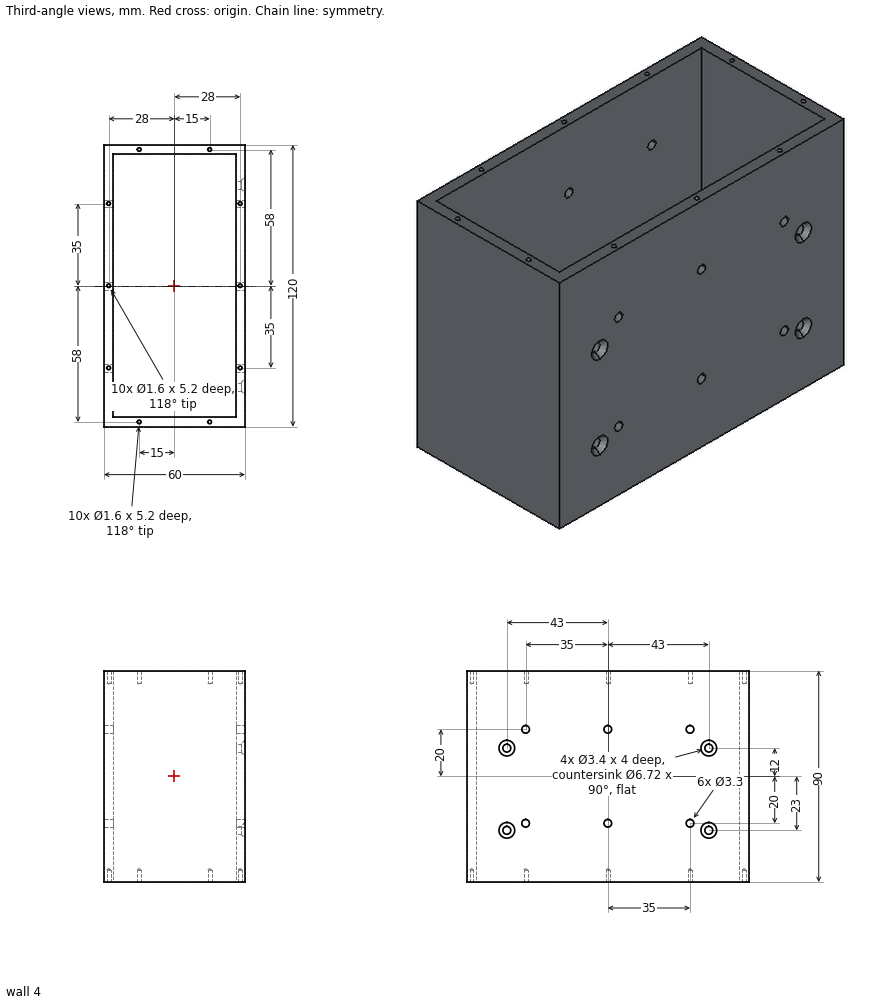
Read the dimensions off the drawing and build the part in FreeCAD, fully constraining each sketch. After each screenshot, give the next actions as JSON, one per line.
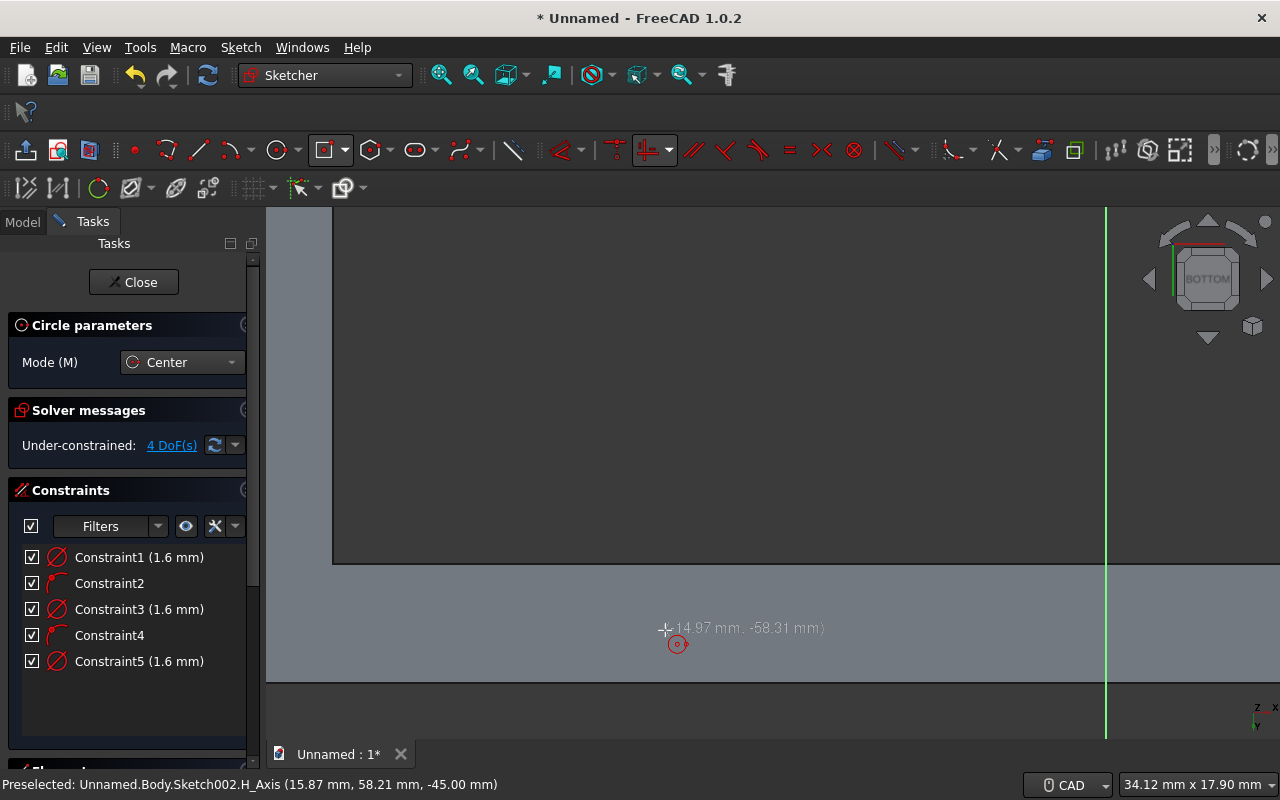
{"action": "scroll", "coordinate": [664, 630], "scroll_direction": "down", "scroll_amount": 12}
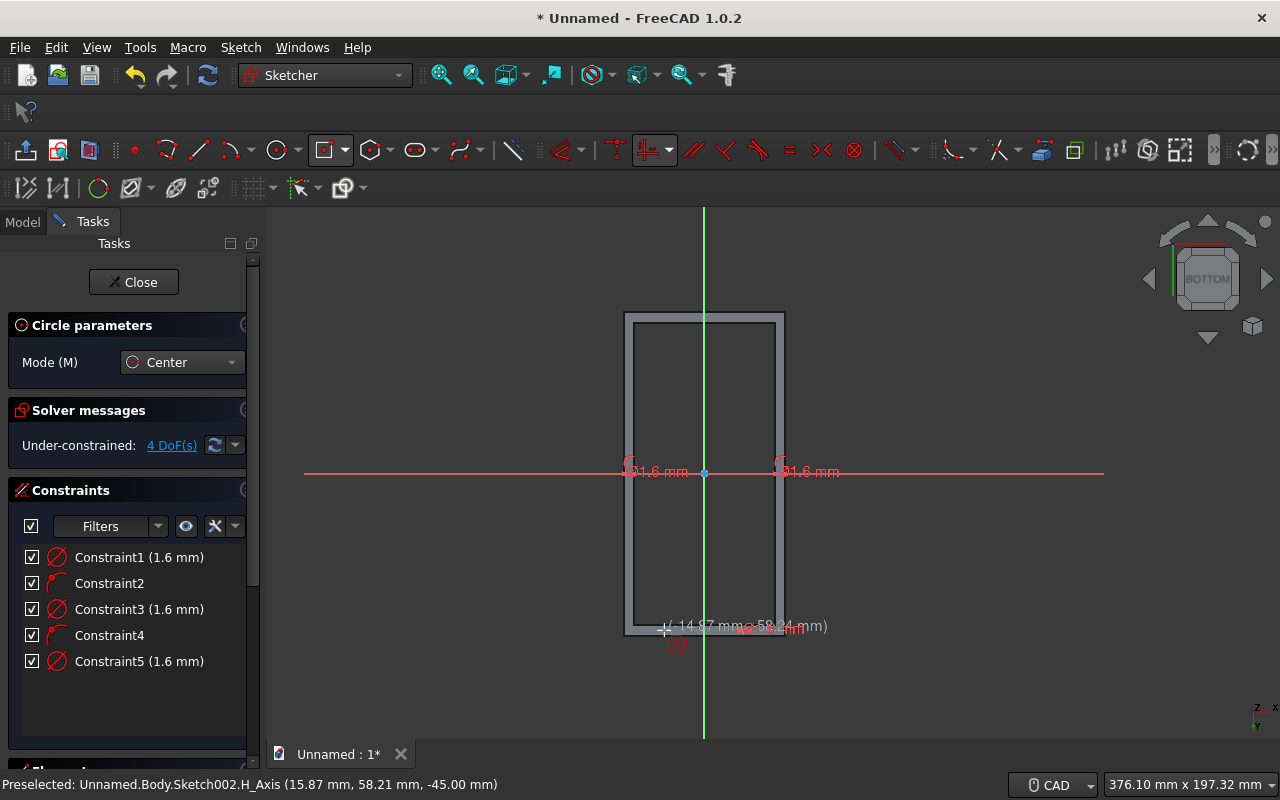
{"action": "left_click", "coordinate": [664, 630]}
{"action": "mouse_move", "coordinate": [666, 629]}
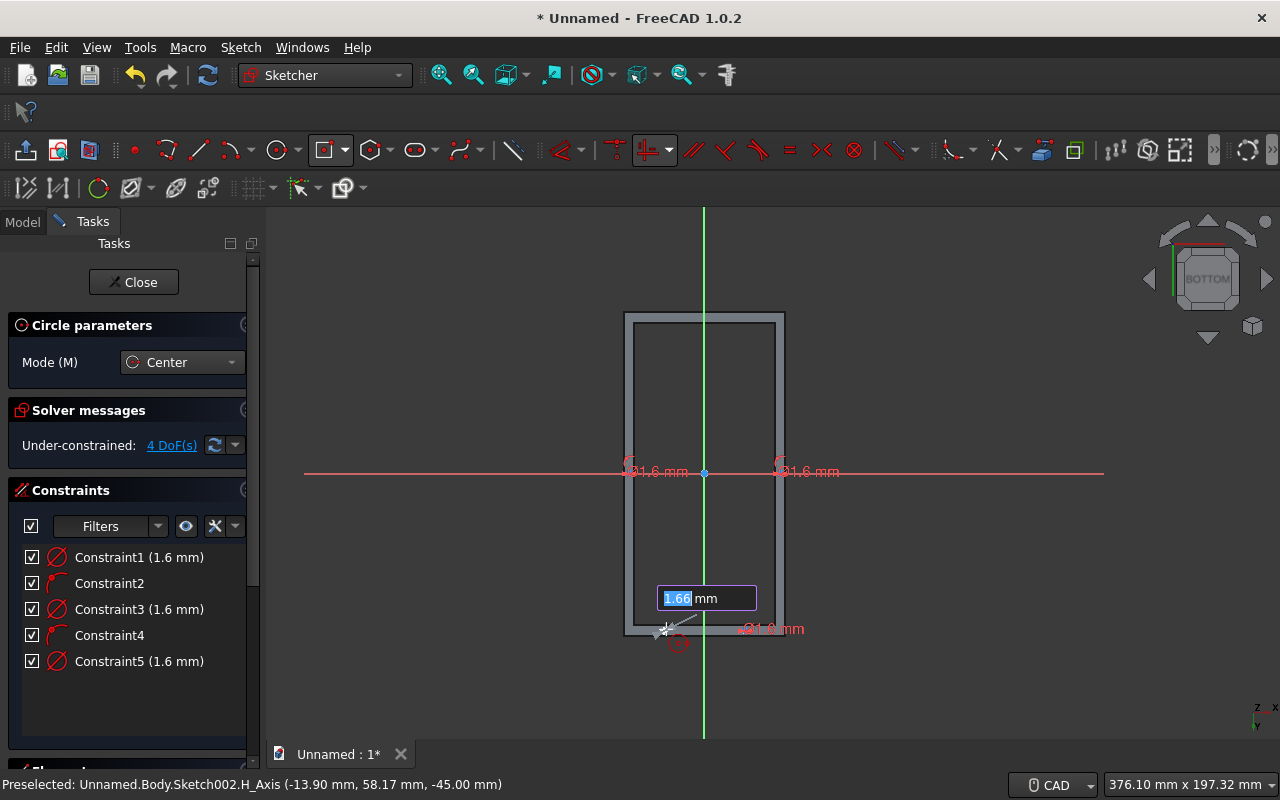
{"action": "type", "text": "1.6"}
{"action": "key", "text": "Return"}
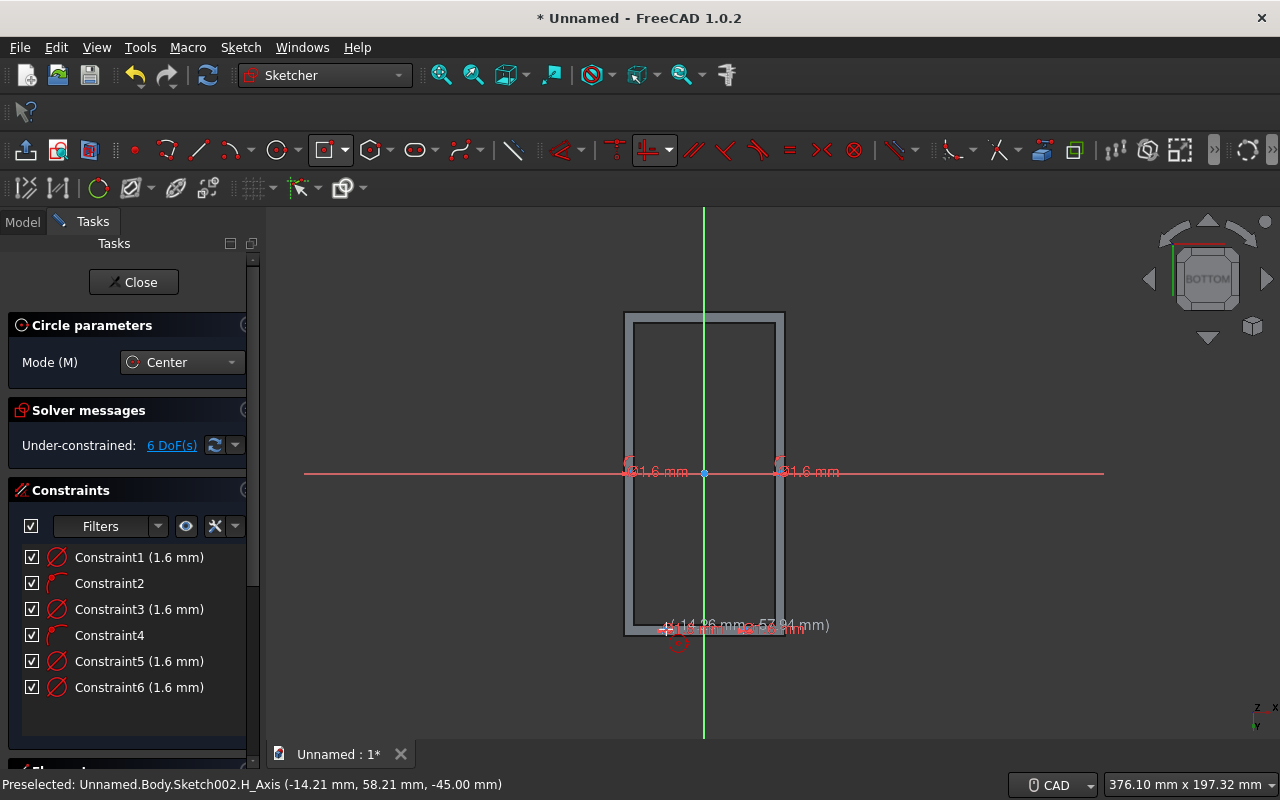
{"action": "scroll", "coordinate": [629, 568], "scroll_direction": "up", "scroll_amount": 12}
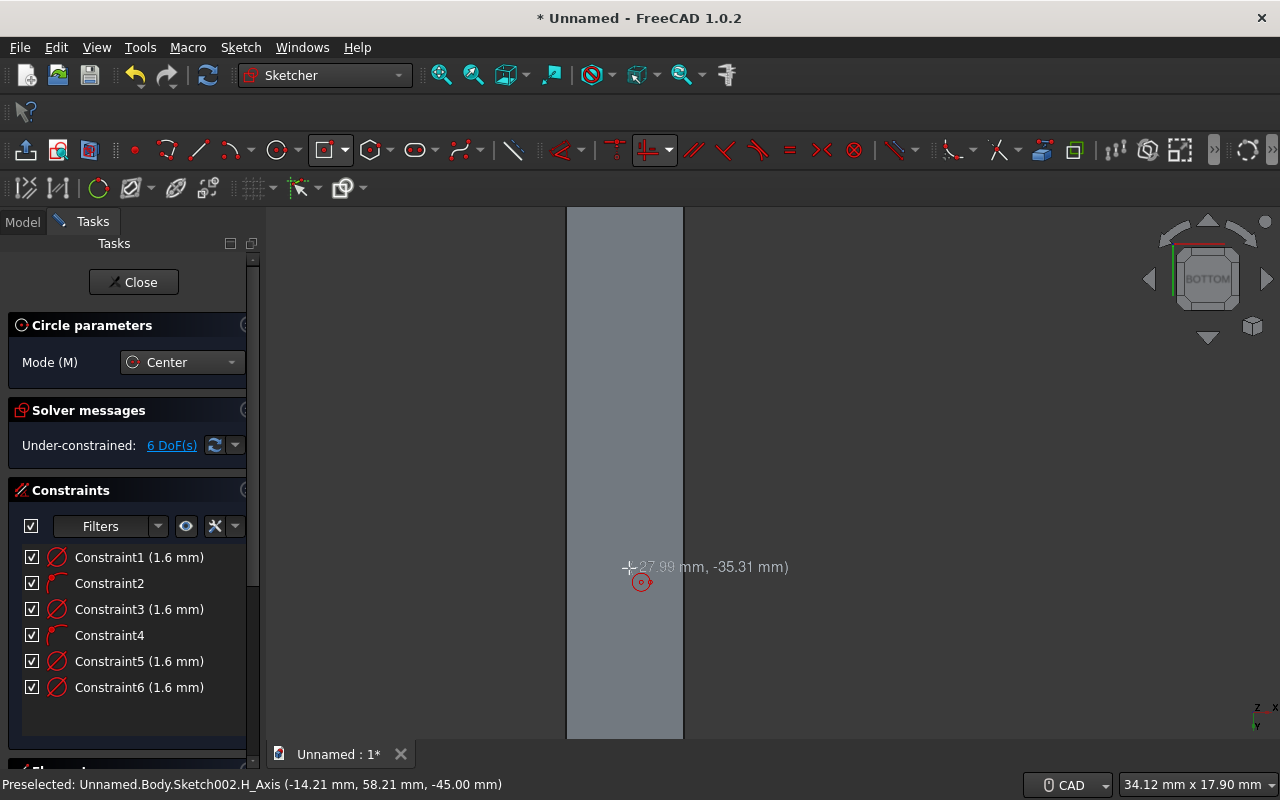
{"action": "scroll", "coordinate": [629, 568], "scroll_direction": "down", "scroll_amount": 12}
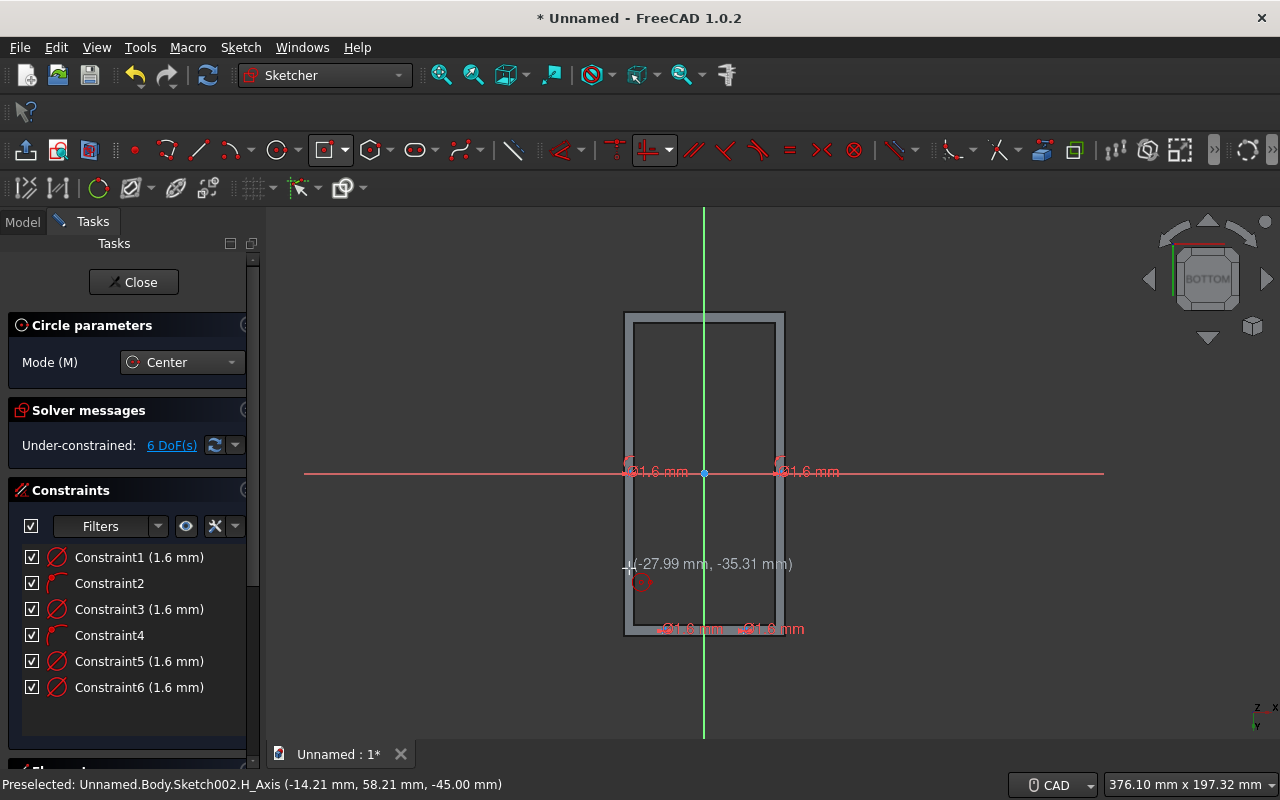
{"action": "left_click", "coordinate": [629, 568]}
{"action": "mouse_move", "coordinate": [630, 567]}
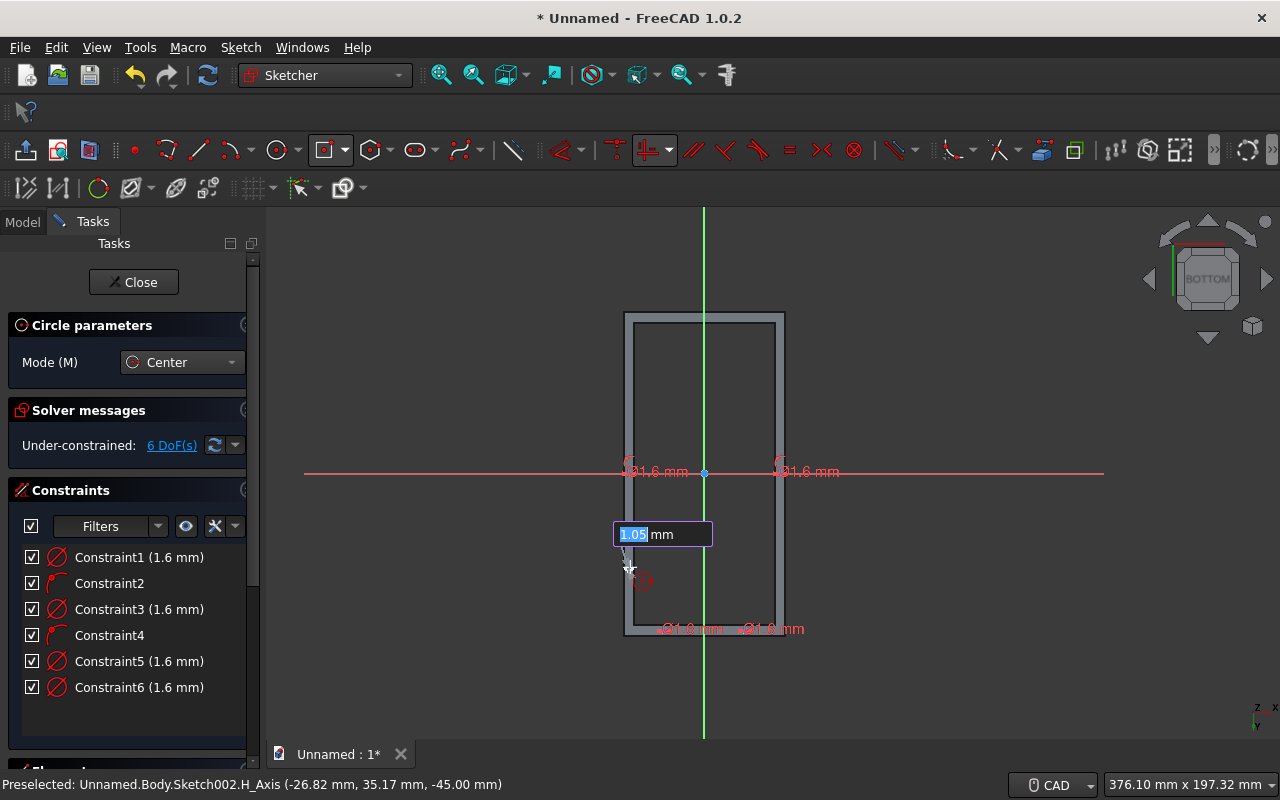
{"action": "type", "text": "1.6"}
{"action": "key", "text": "Return"}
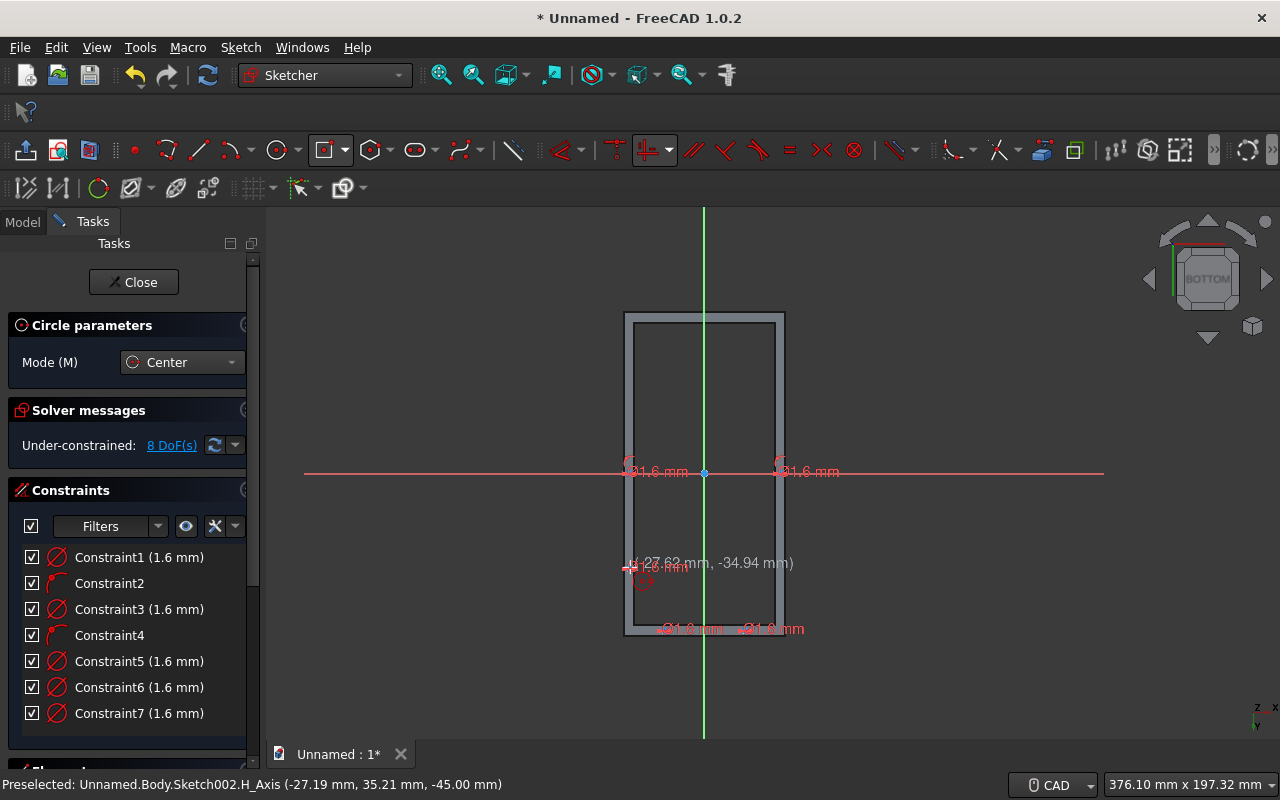
{"action": "scroll", "coordinate": [780, 568], "scroll_direction": "up", "scroll_amount": 12}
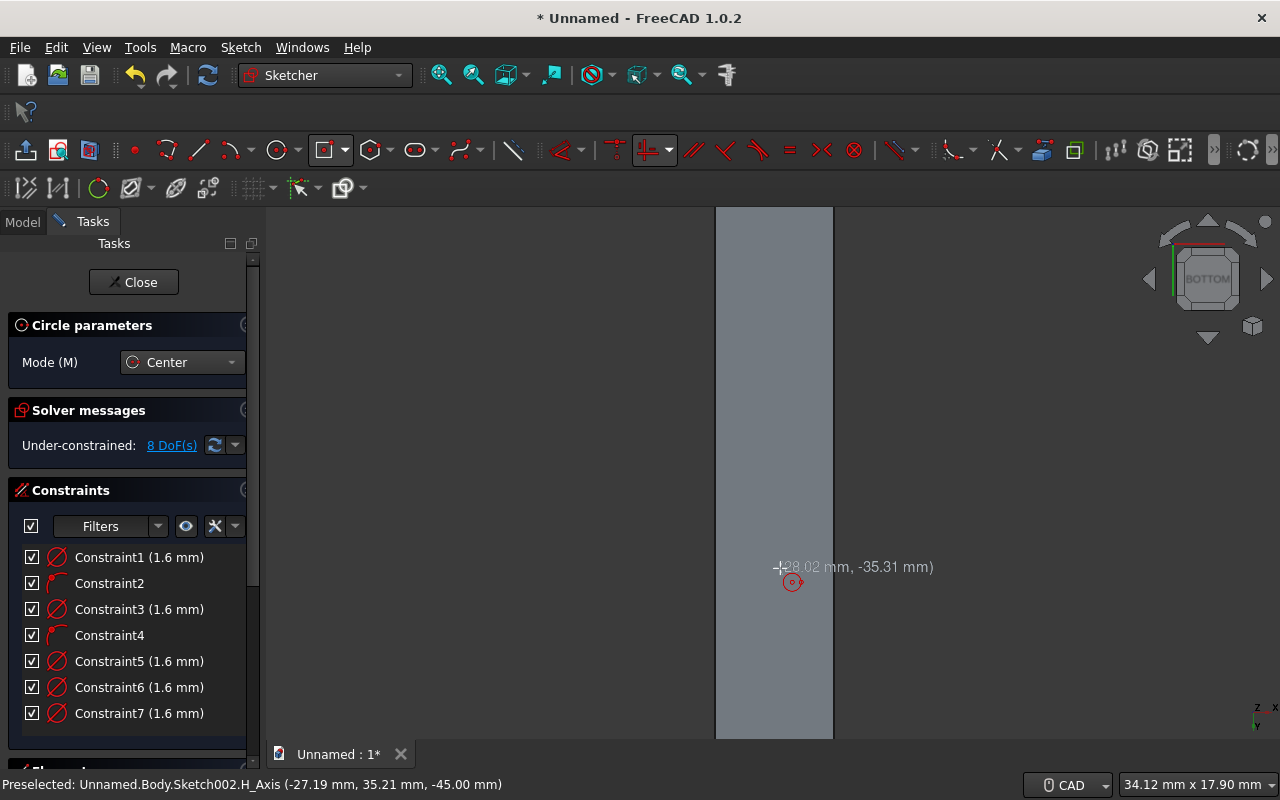
{"action": "scroll", "coordinate": [781, 568], "scroll_direction": "down", "scroll_amount": 12}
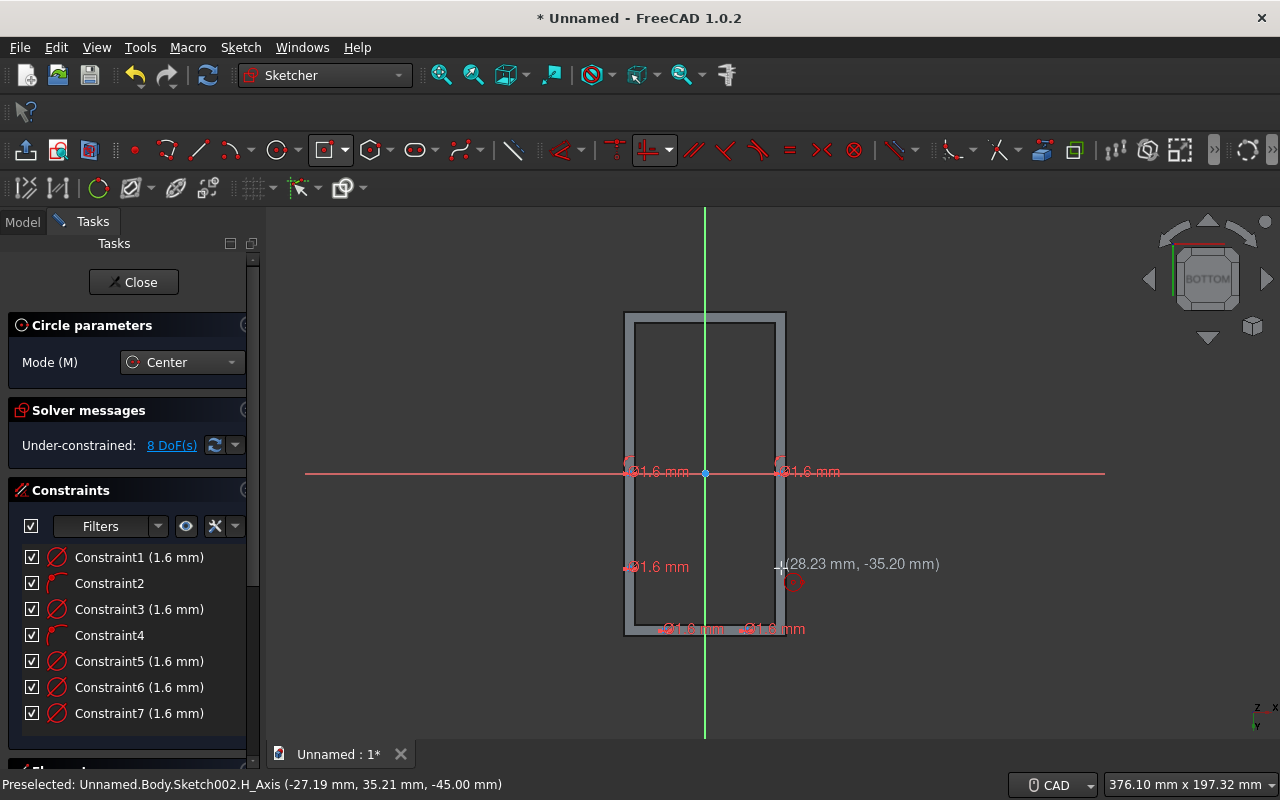
{"action": "left_click", "coordinate": [781, 568]}
{"action": "mouse_move", "coordinate": [782, 567]}